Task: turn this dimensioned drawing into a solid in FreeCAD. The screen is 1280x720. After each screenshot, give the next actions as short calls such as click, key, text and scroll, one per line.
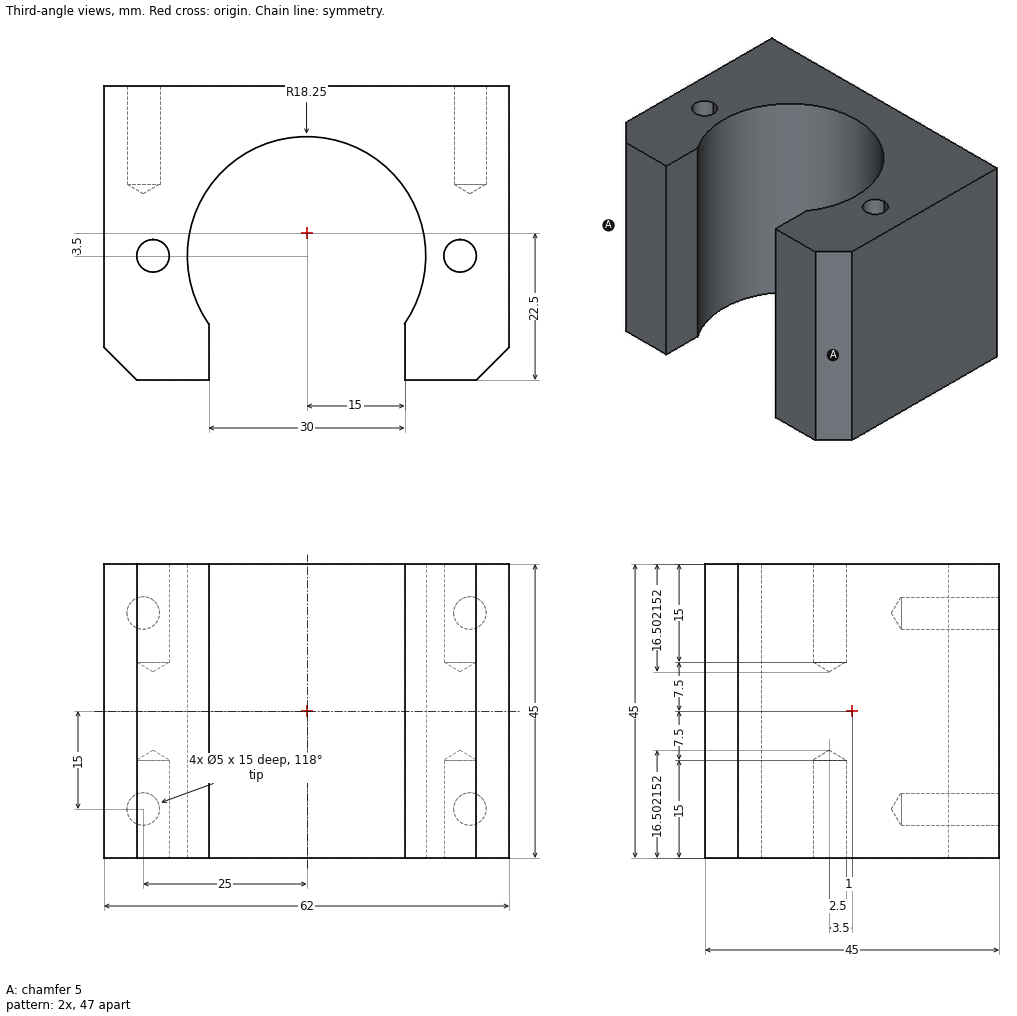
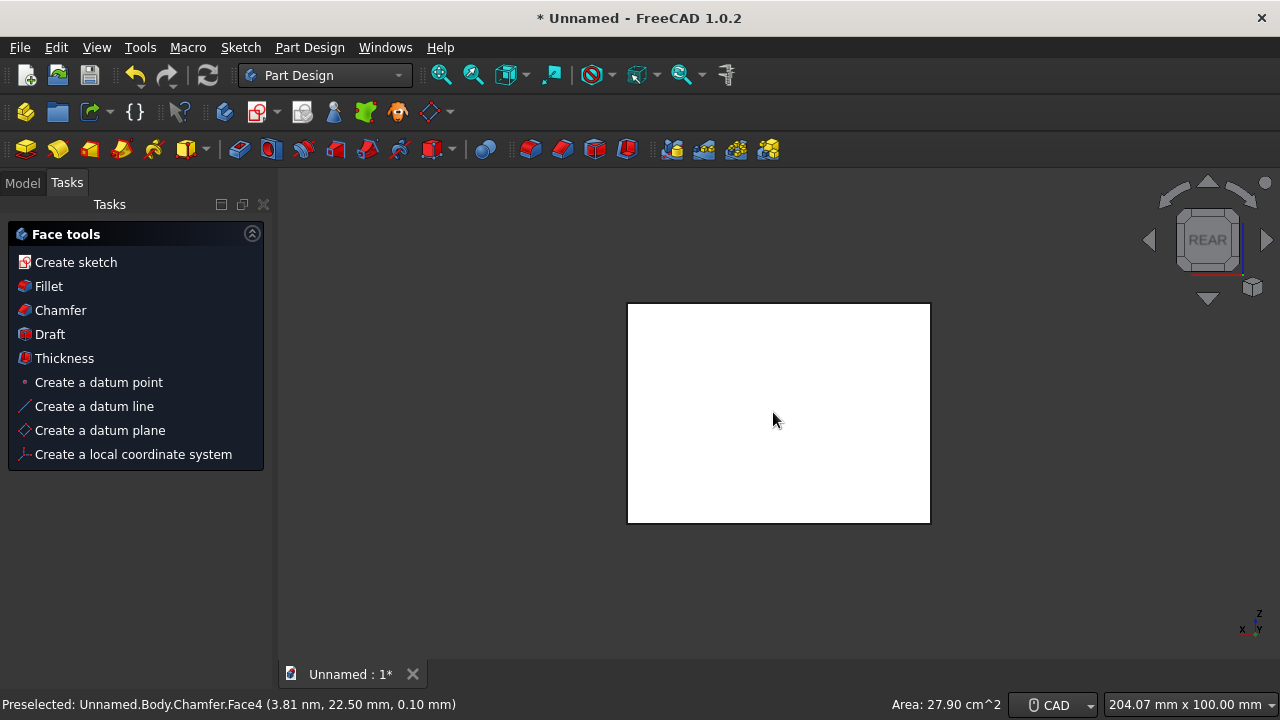
click(258, 112)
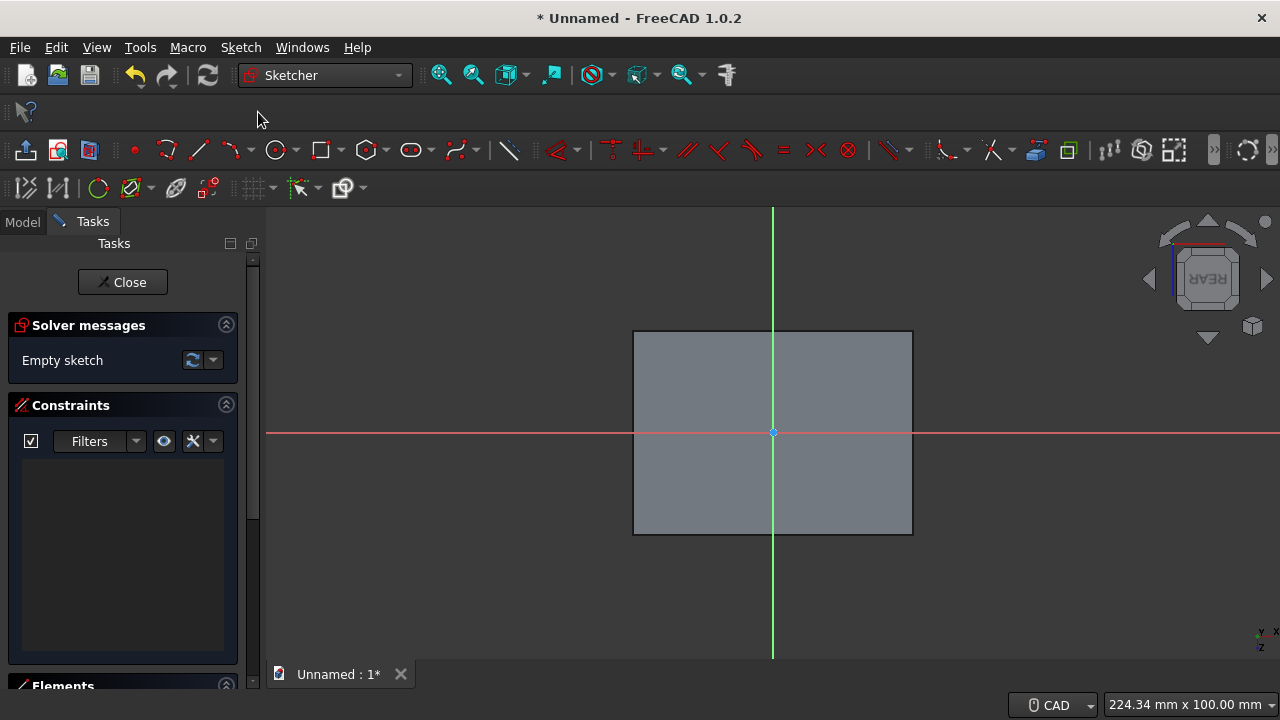
scroll(856, 433, up, 3)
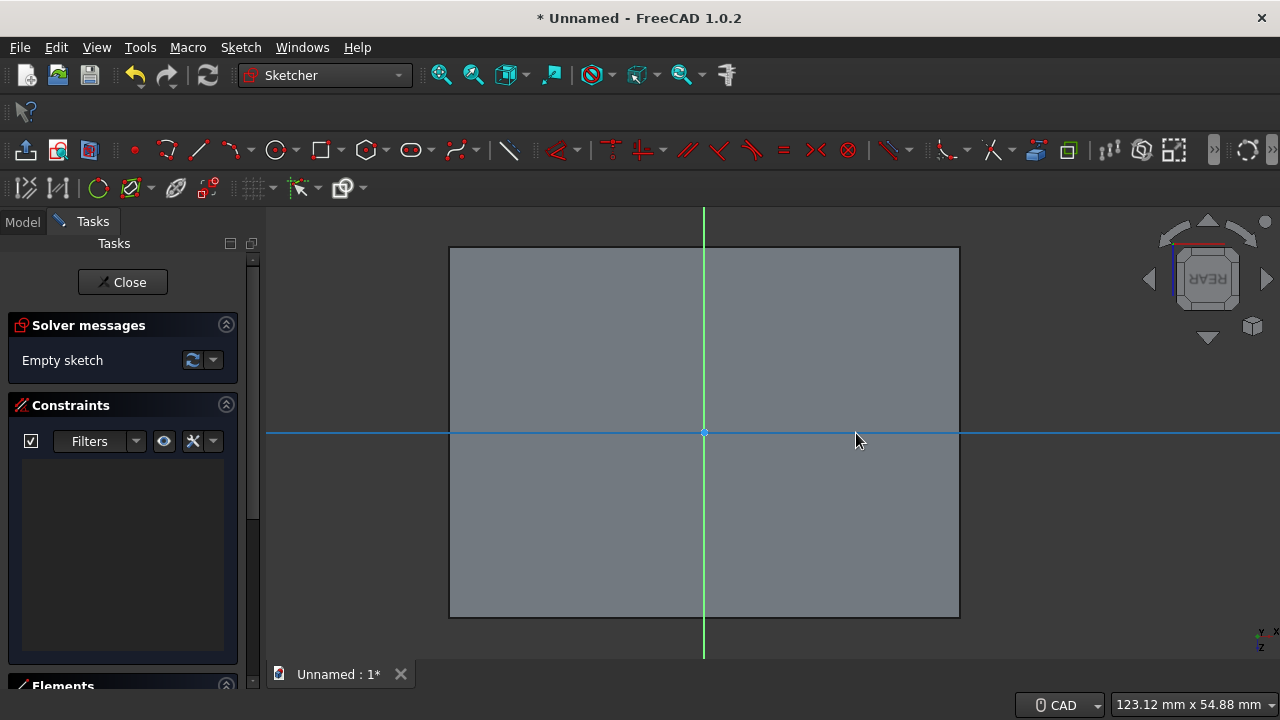
click(276, 150)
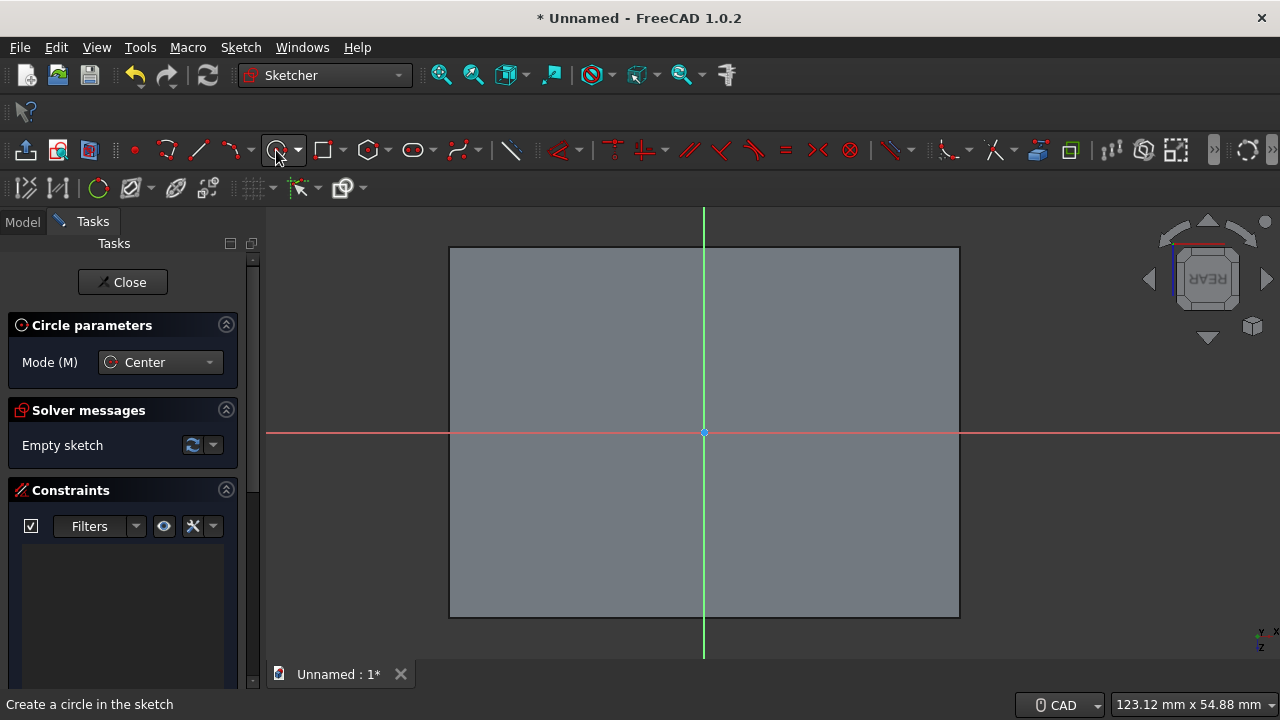
click(498, 309)
click(513, 294)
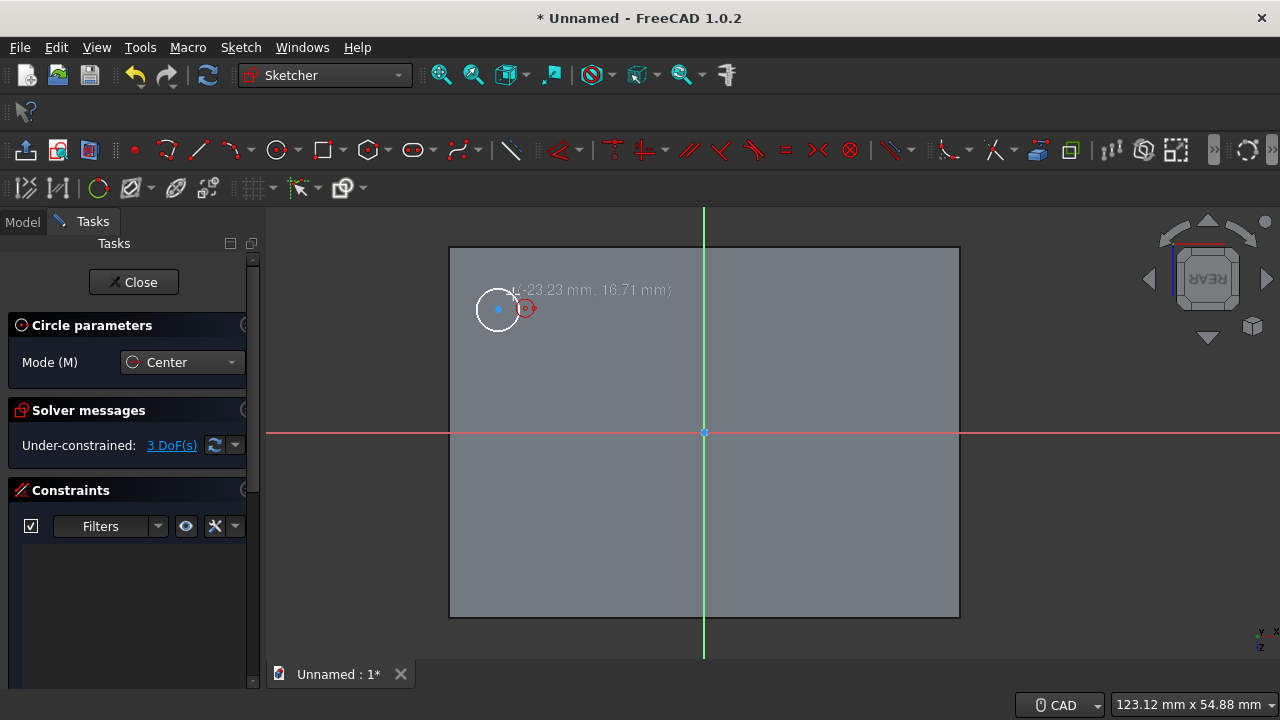
click(498, 556)
click(513, 542)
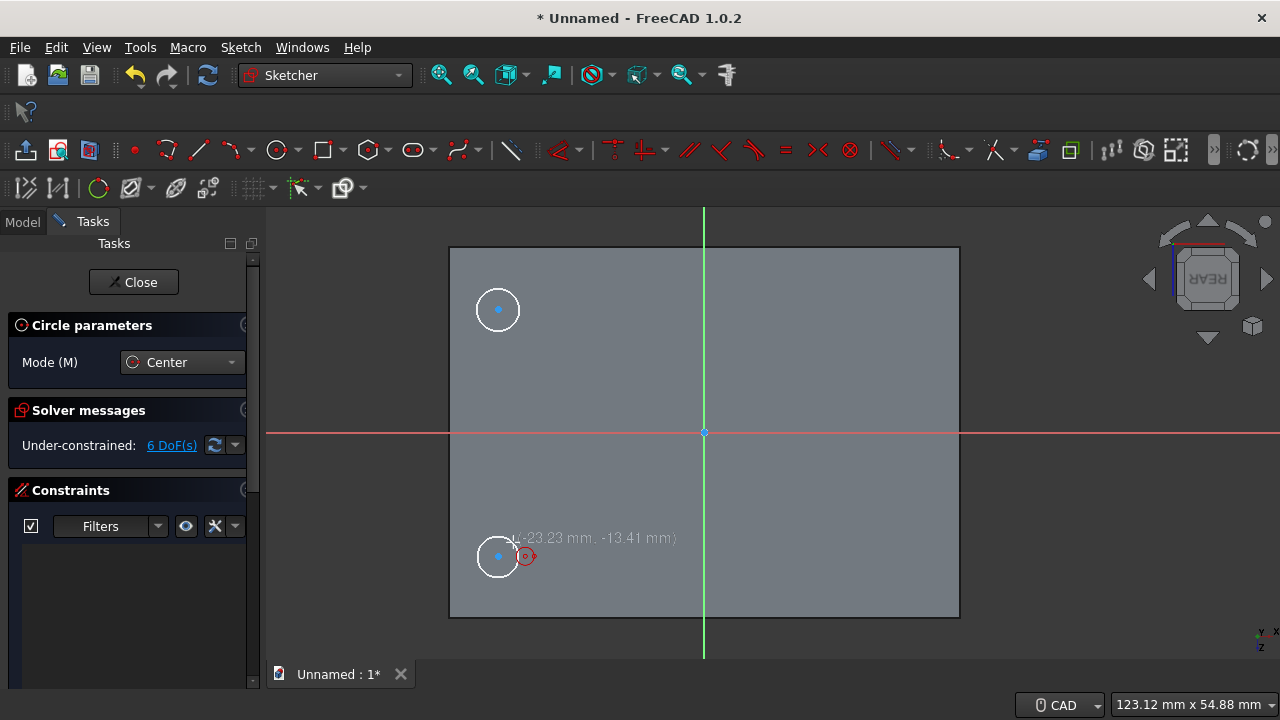
click(910, 556)
click(925, 542)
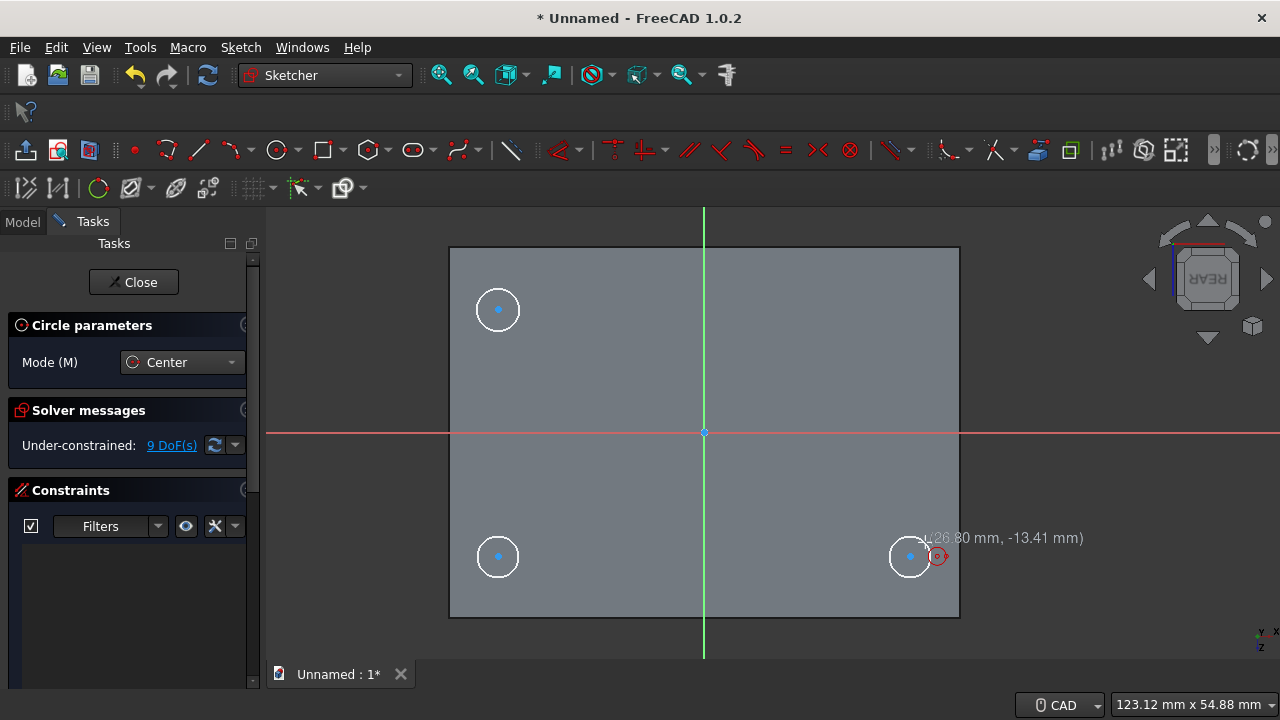
click(910, 309)
click(925, 294)
key(Escape)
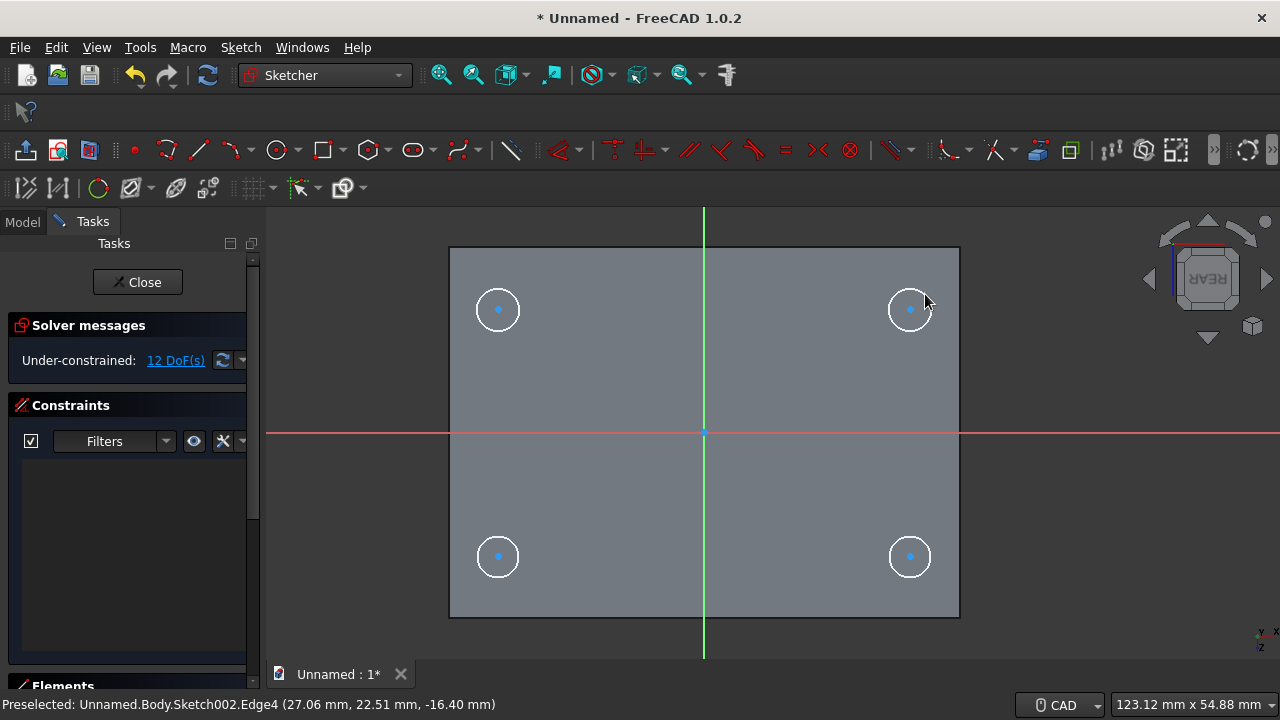
click(513, 295)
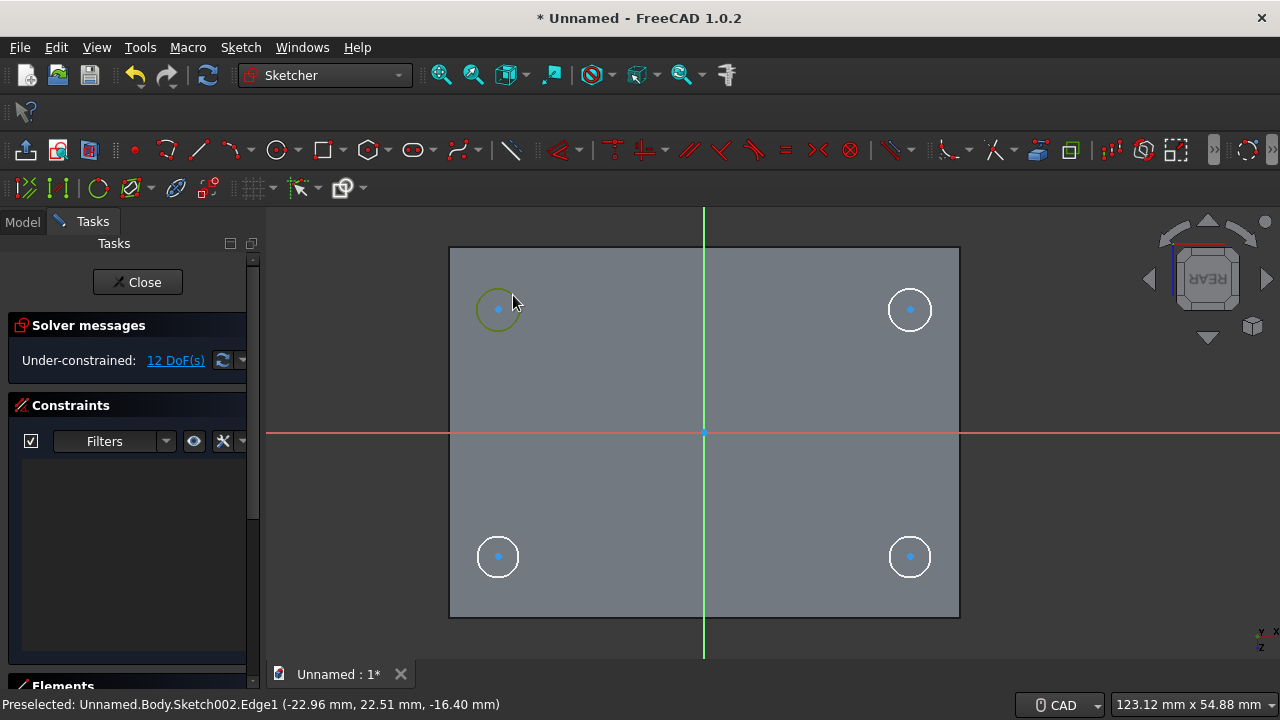
click(512, 542)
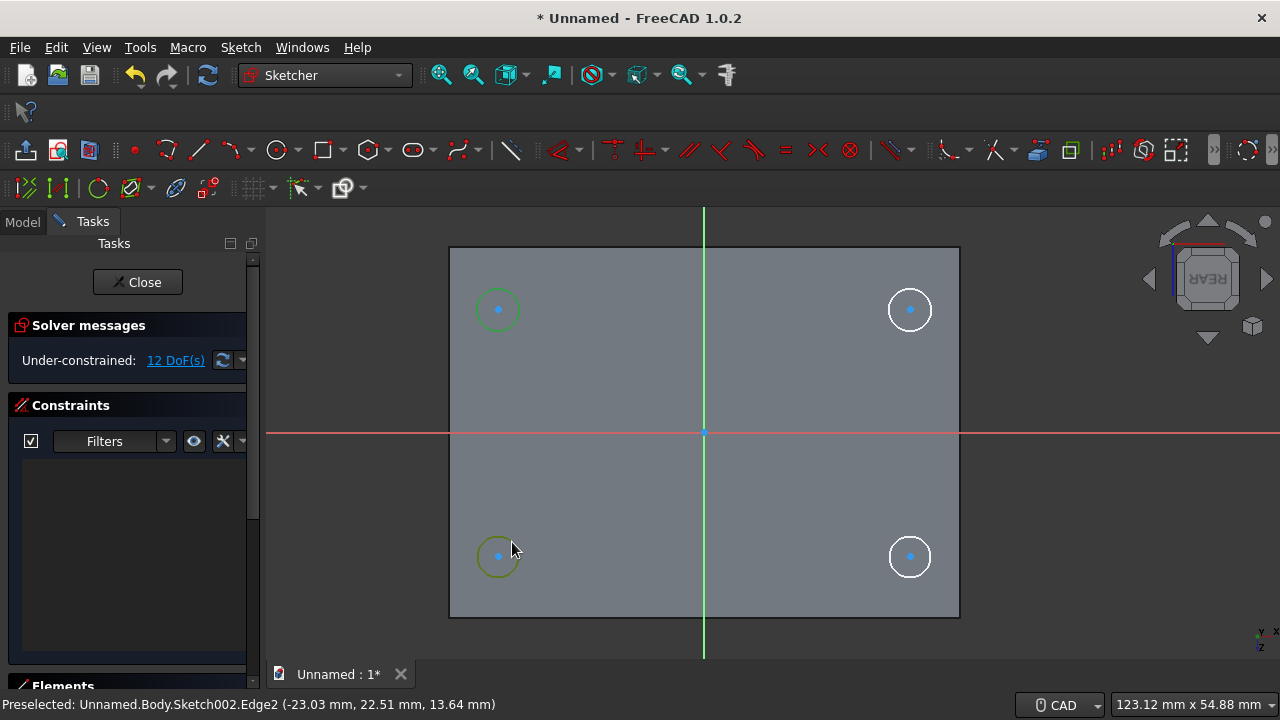
click(924, 542)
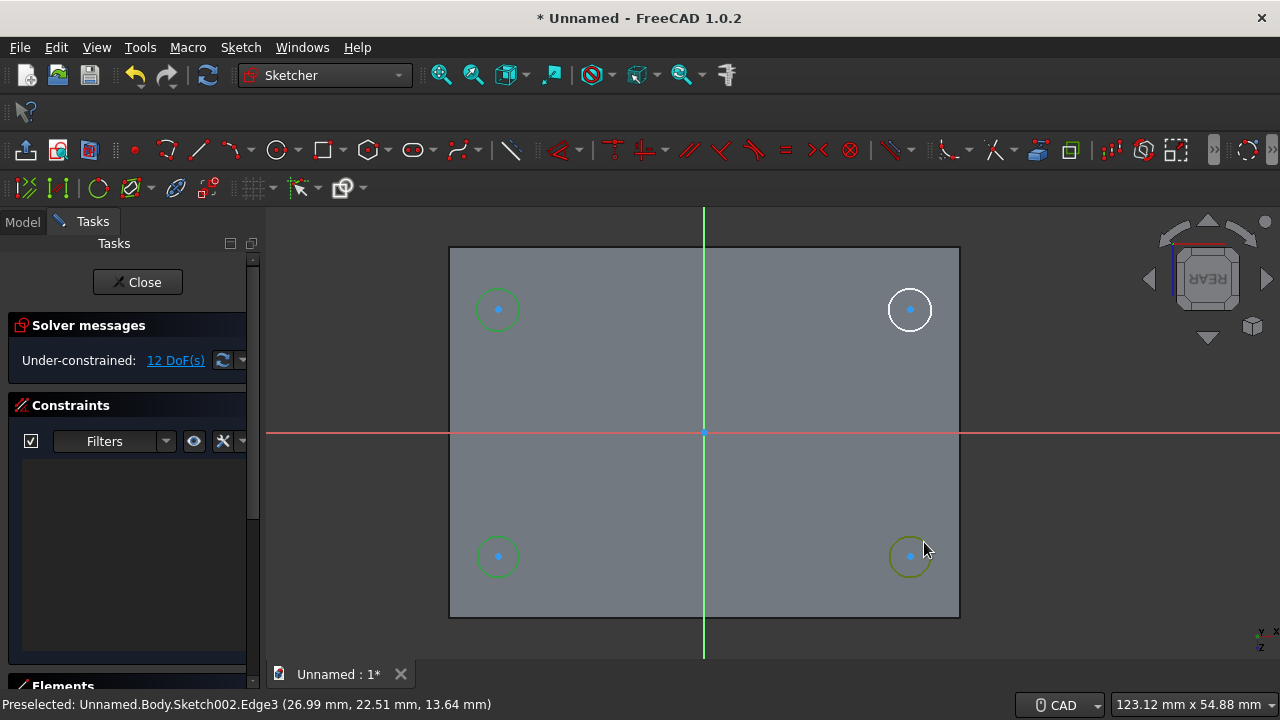
click(925, 295)